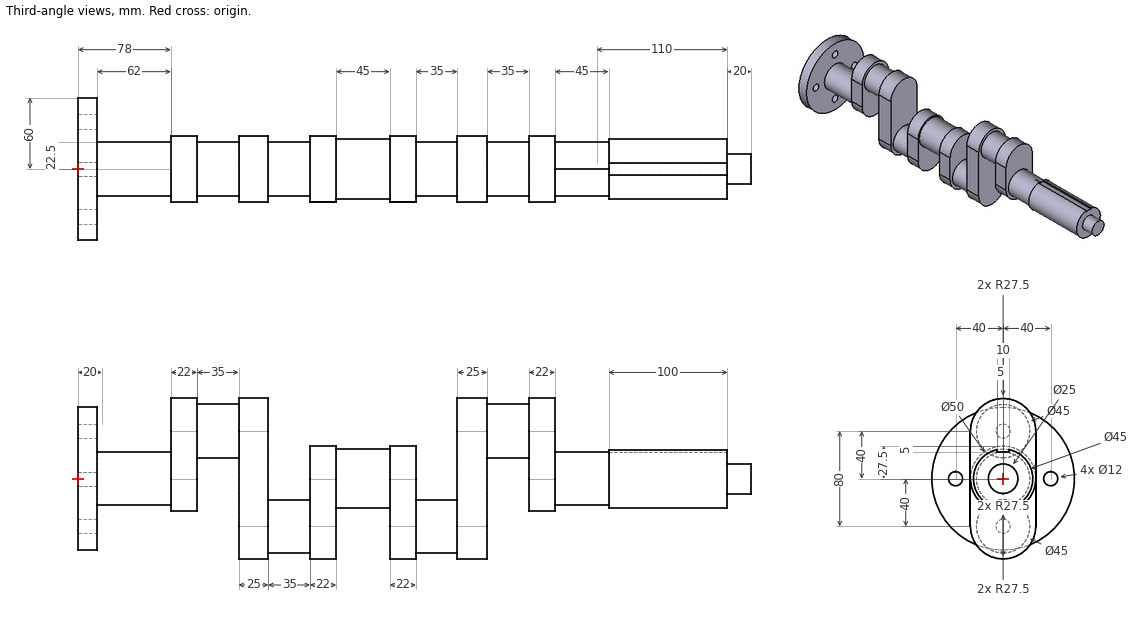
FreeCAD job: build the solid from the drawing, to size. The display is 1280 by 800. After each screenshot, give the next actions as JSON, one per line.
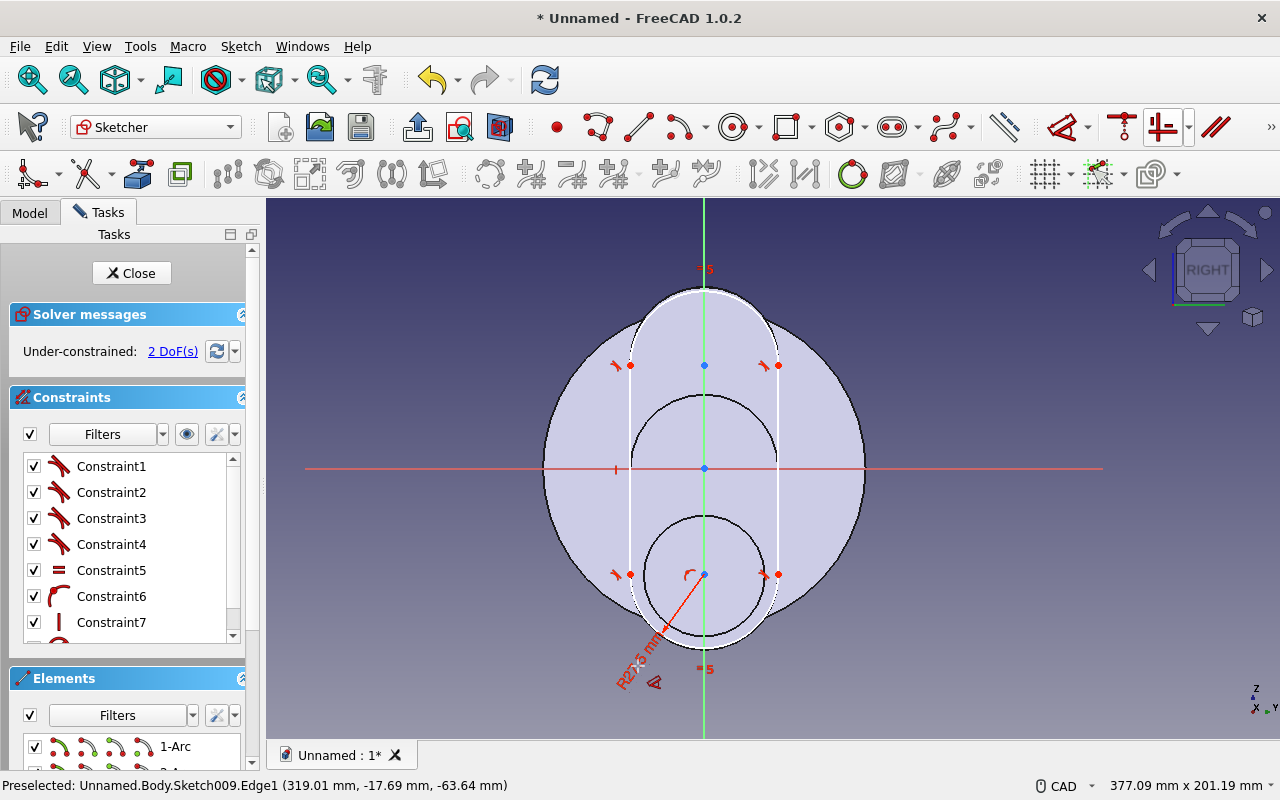
{"action": "left_click", "coordinate": [630, 511]}
{"action": "left_click", "coordinate": [596, 422]}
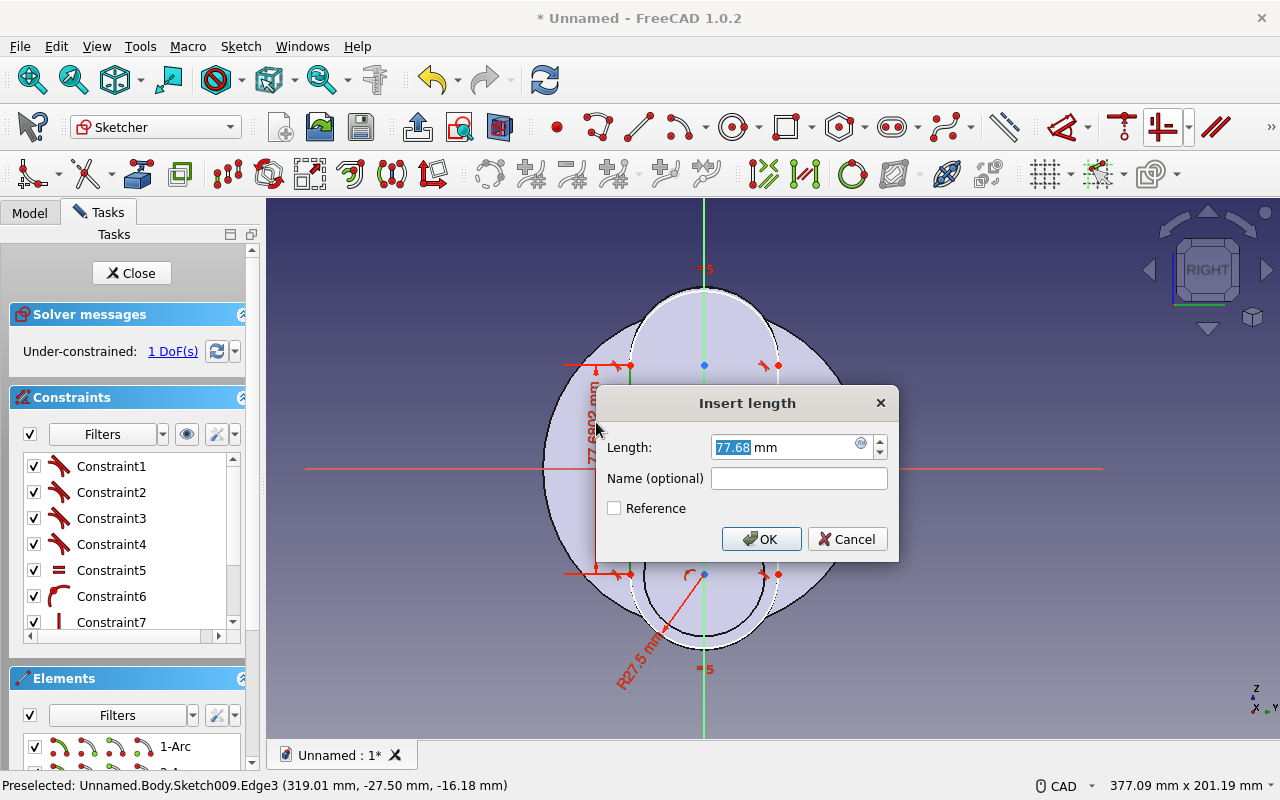
{"action": "type", "text": "80"}
{"action": "key", "text": "Return"}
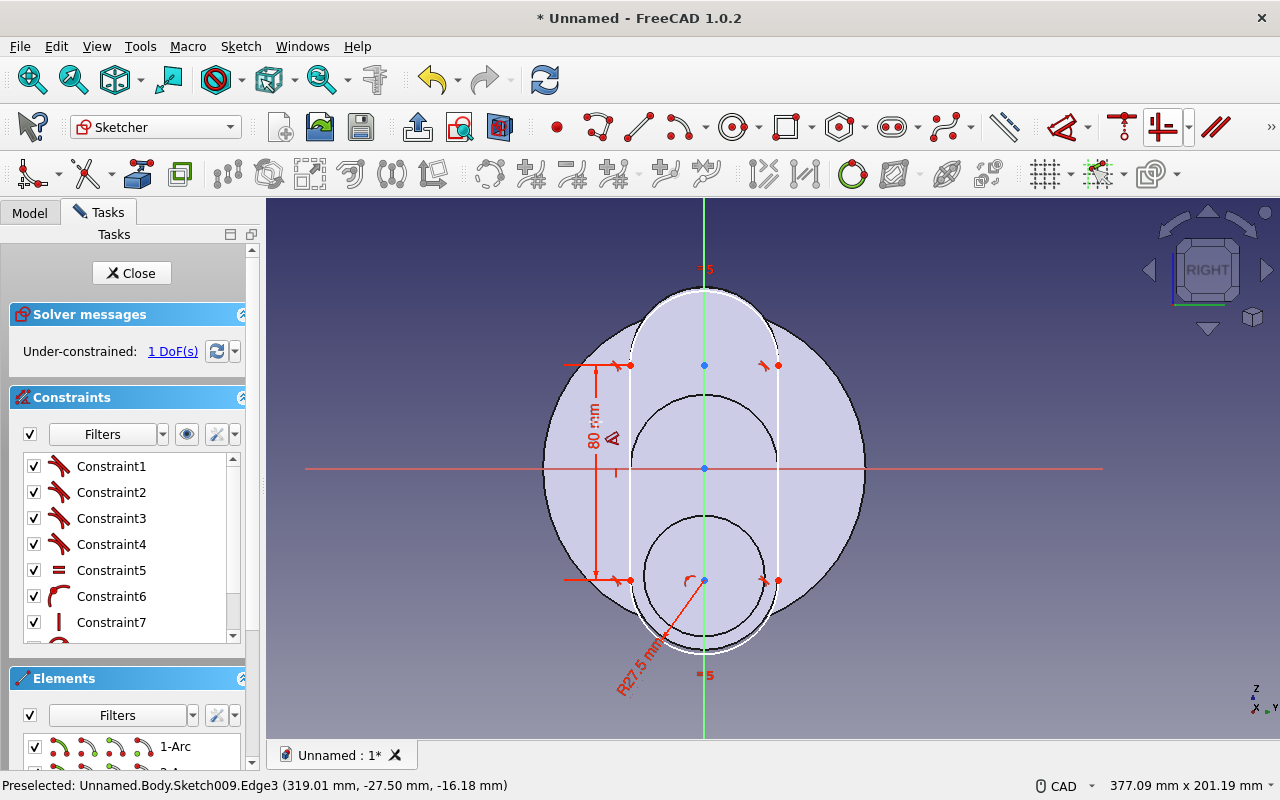
{"action": "left_click", "coordinate": [630, 580]}
{"action": "left_click", "coordinate": [596, 524]}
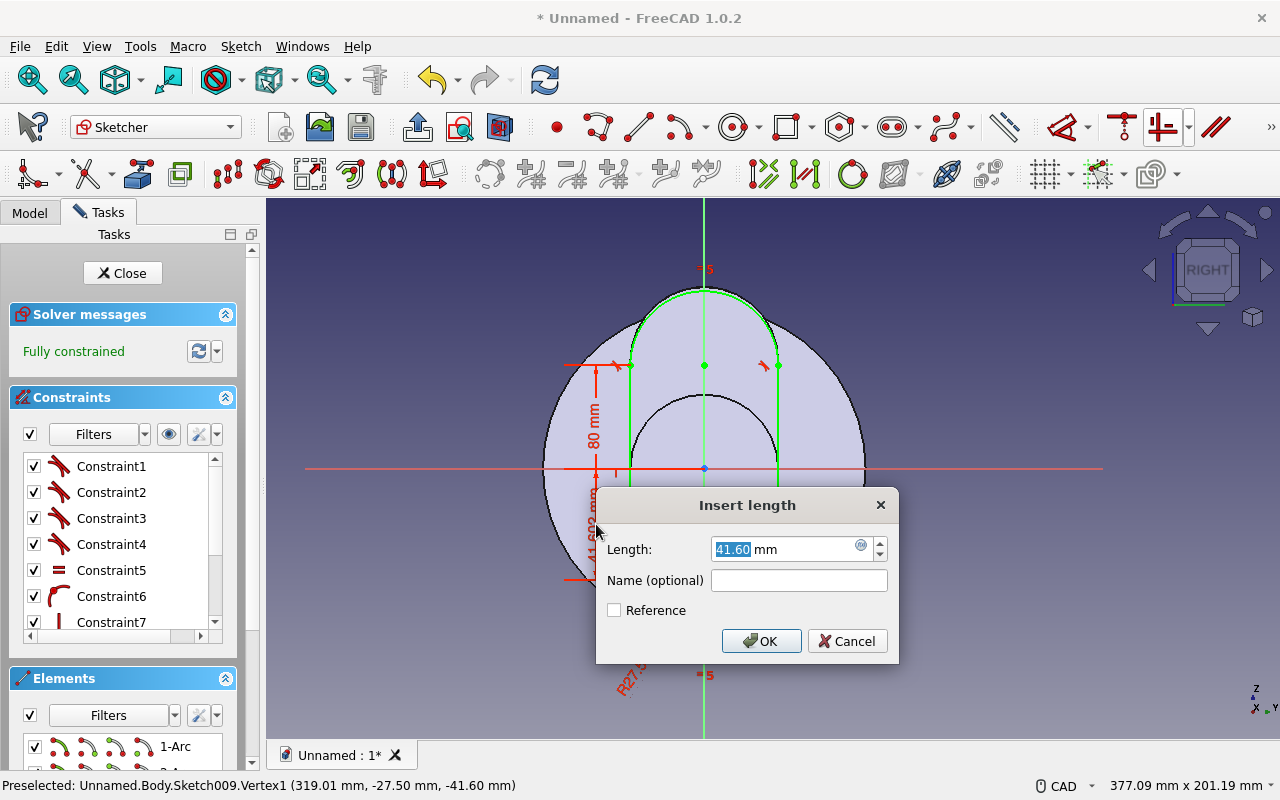
{"action": "type", "text": "40"}
{"action": "key", "text": "Return"}
{"action": "key", "text": "Escape"}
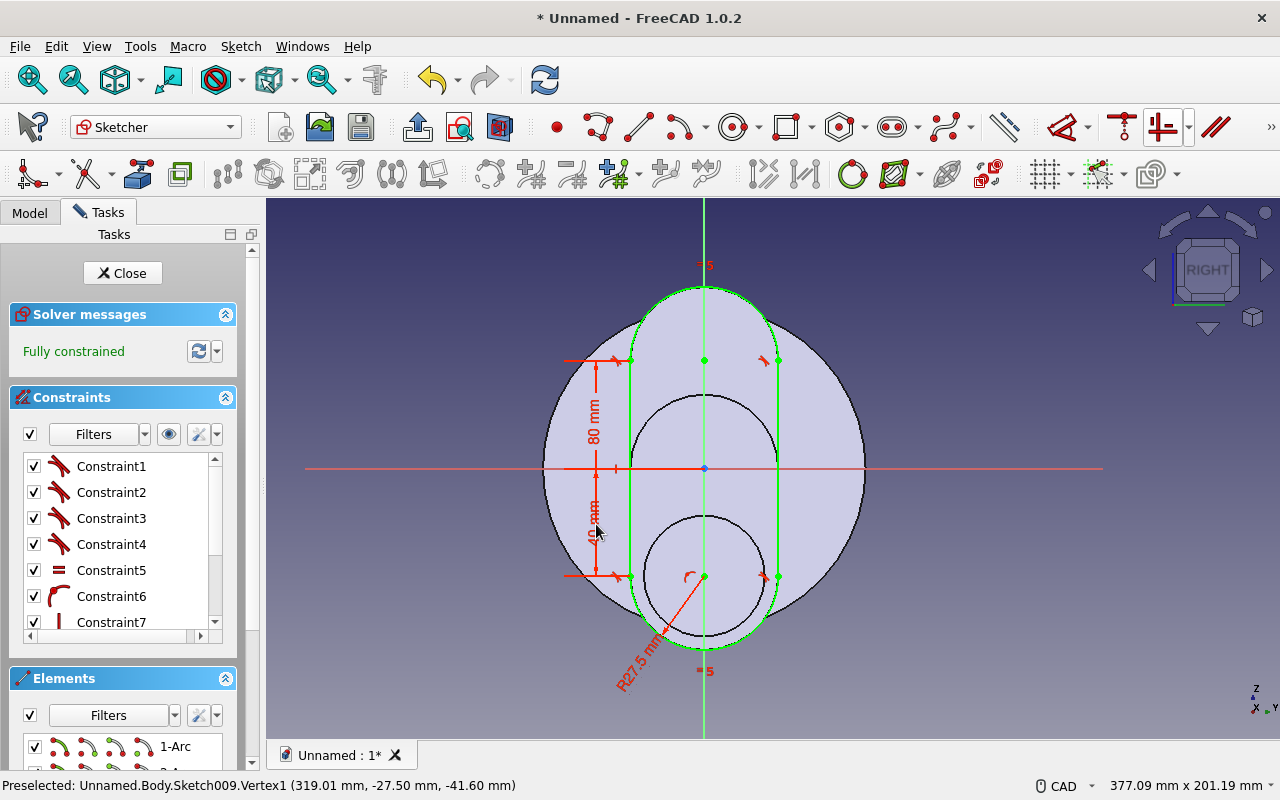
{"action": "left_click", "coordinate": [123, 273]}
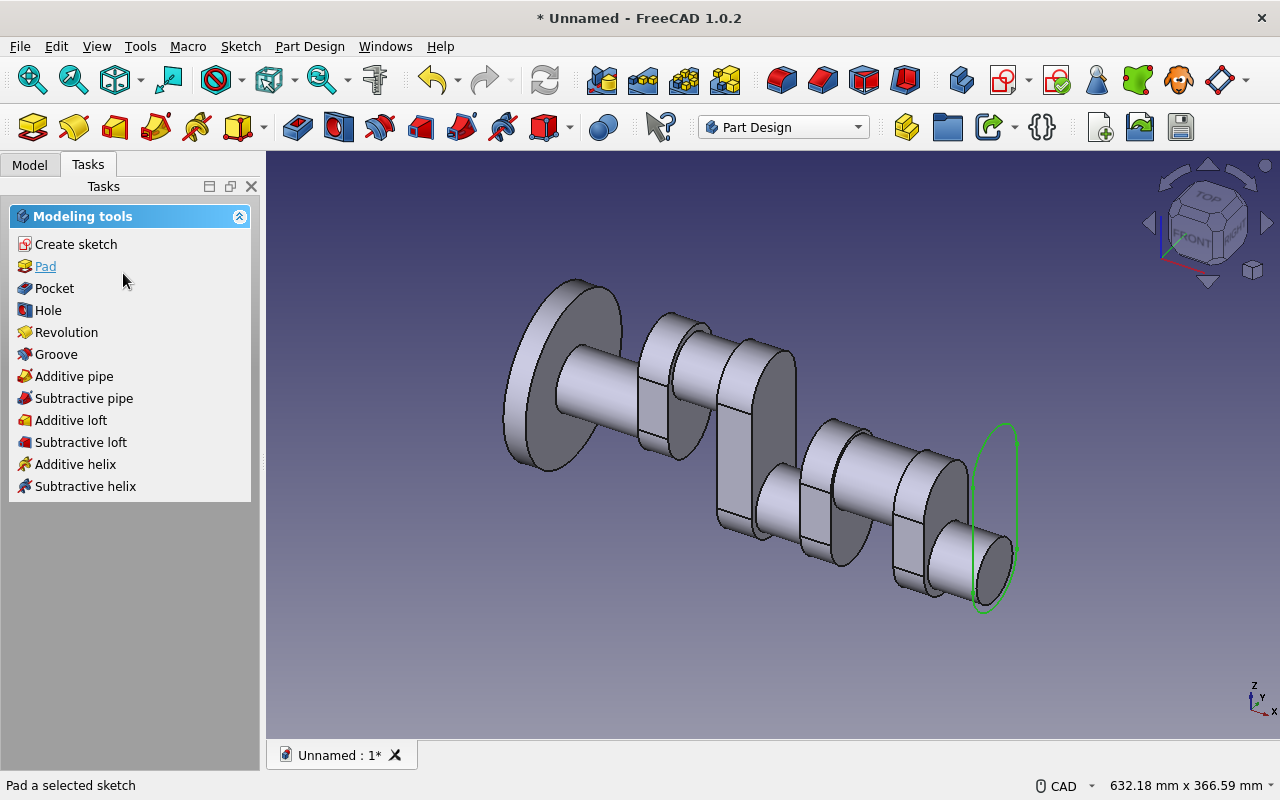
{"action": "left_click", "coordinate": [33, 128]}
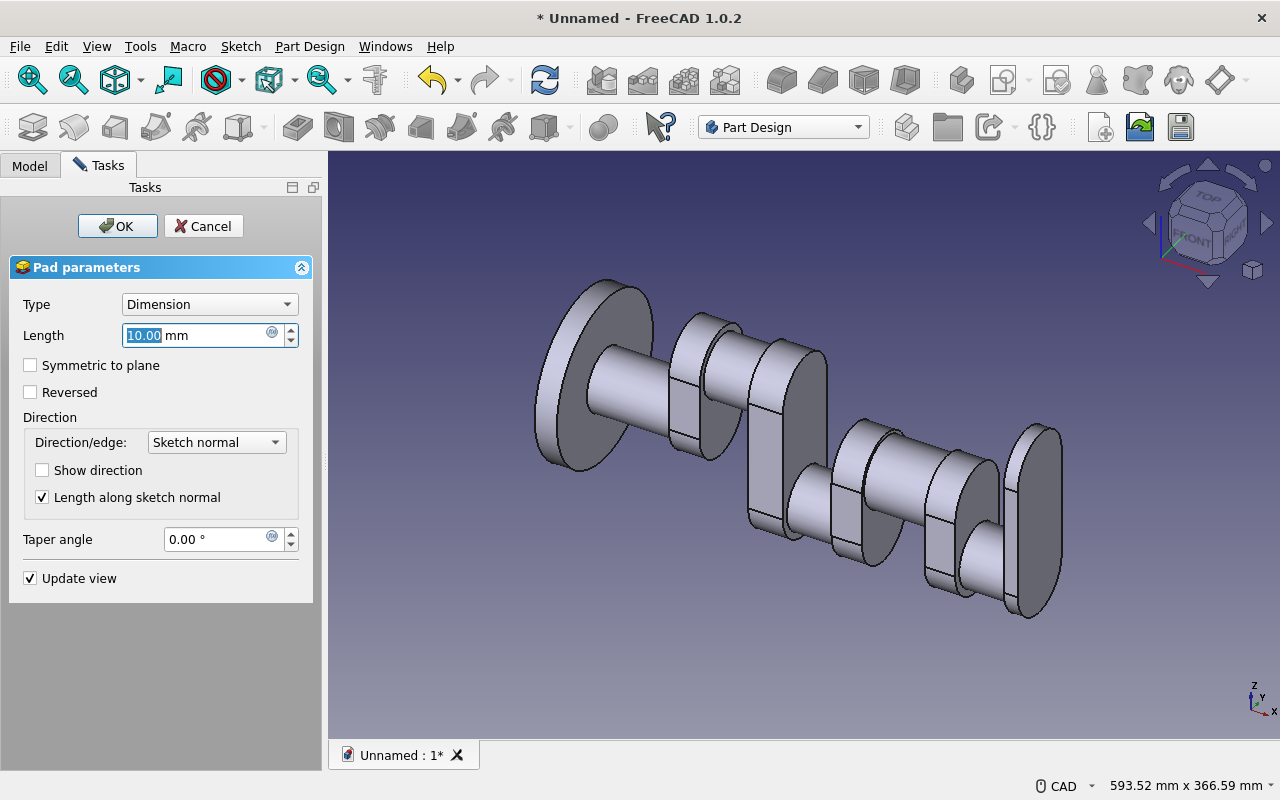
{"action": "type", "text": "25"}
{"action": "key", "text": "Tab"}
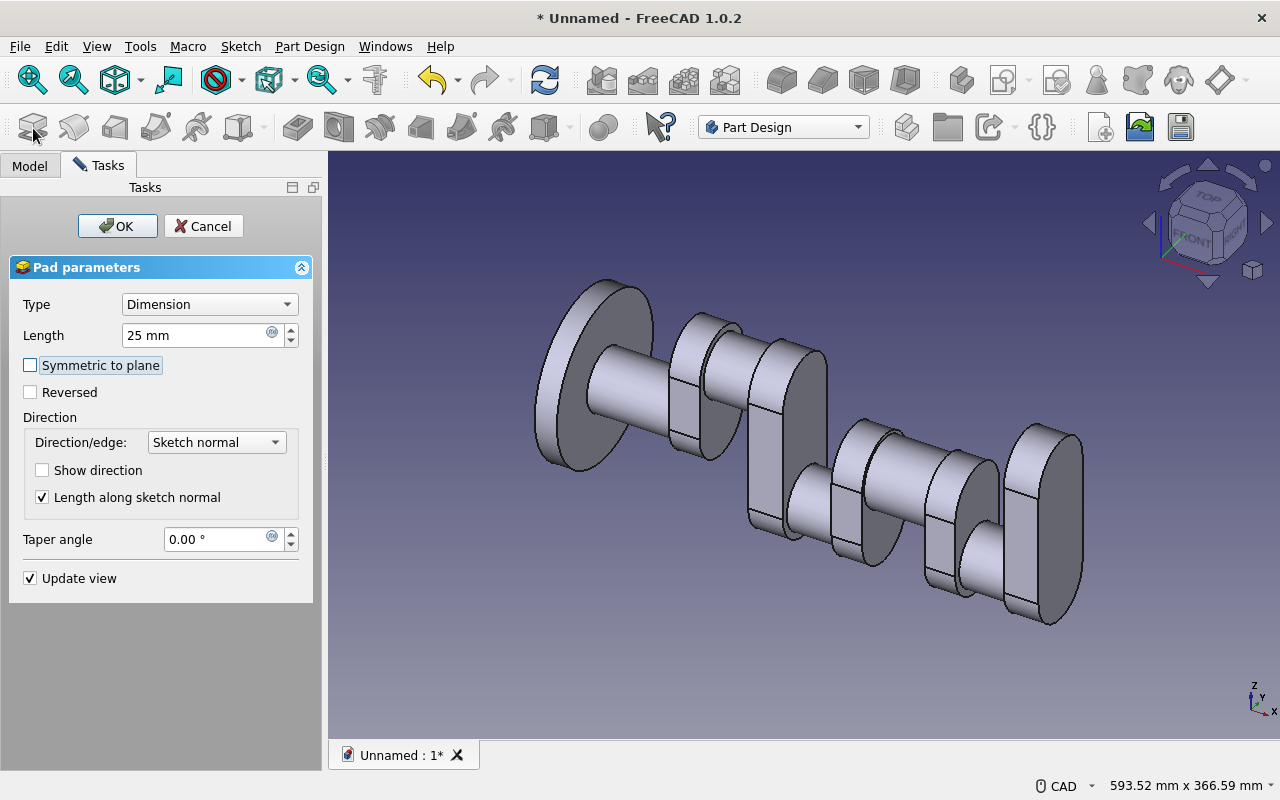
{"action": "left_click", "coordinate": [118, 226]}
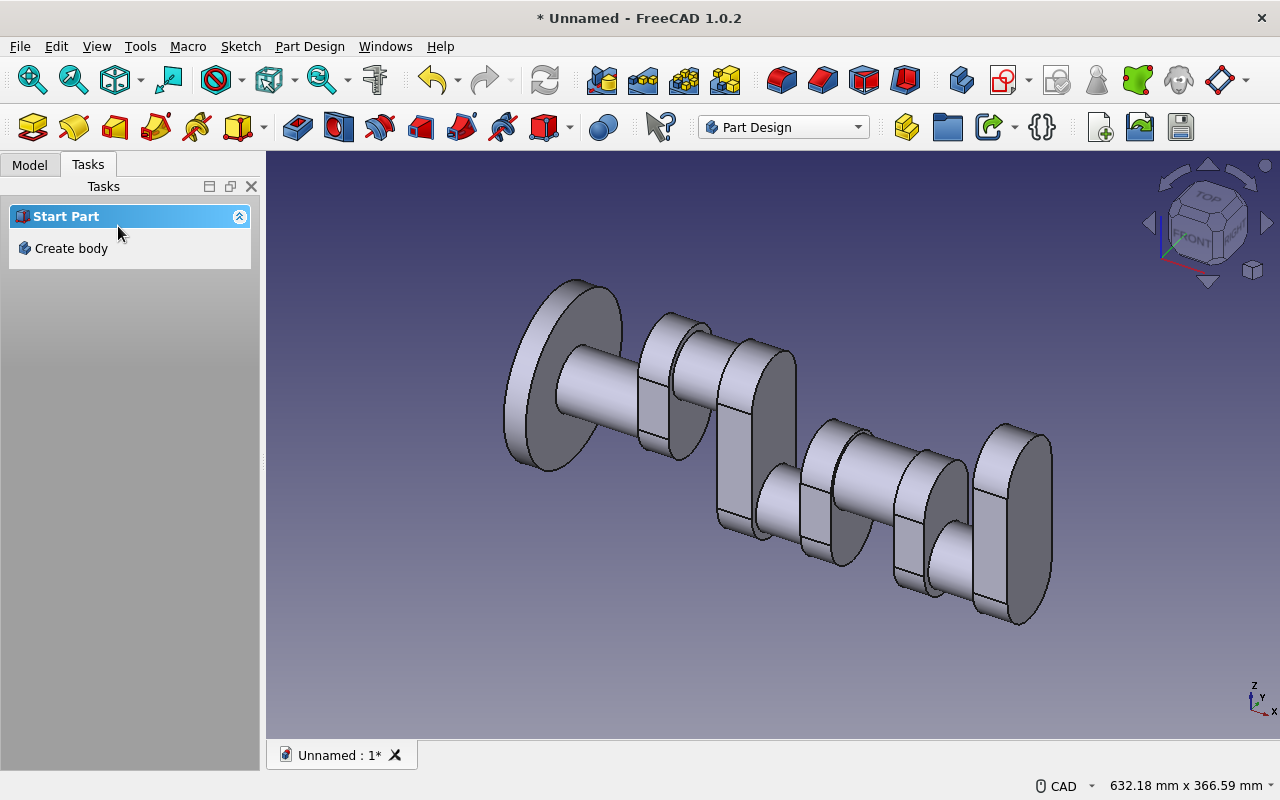
{"action": "left_click", "coordinate": [1030, 478]}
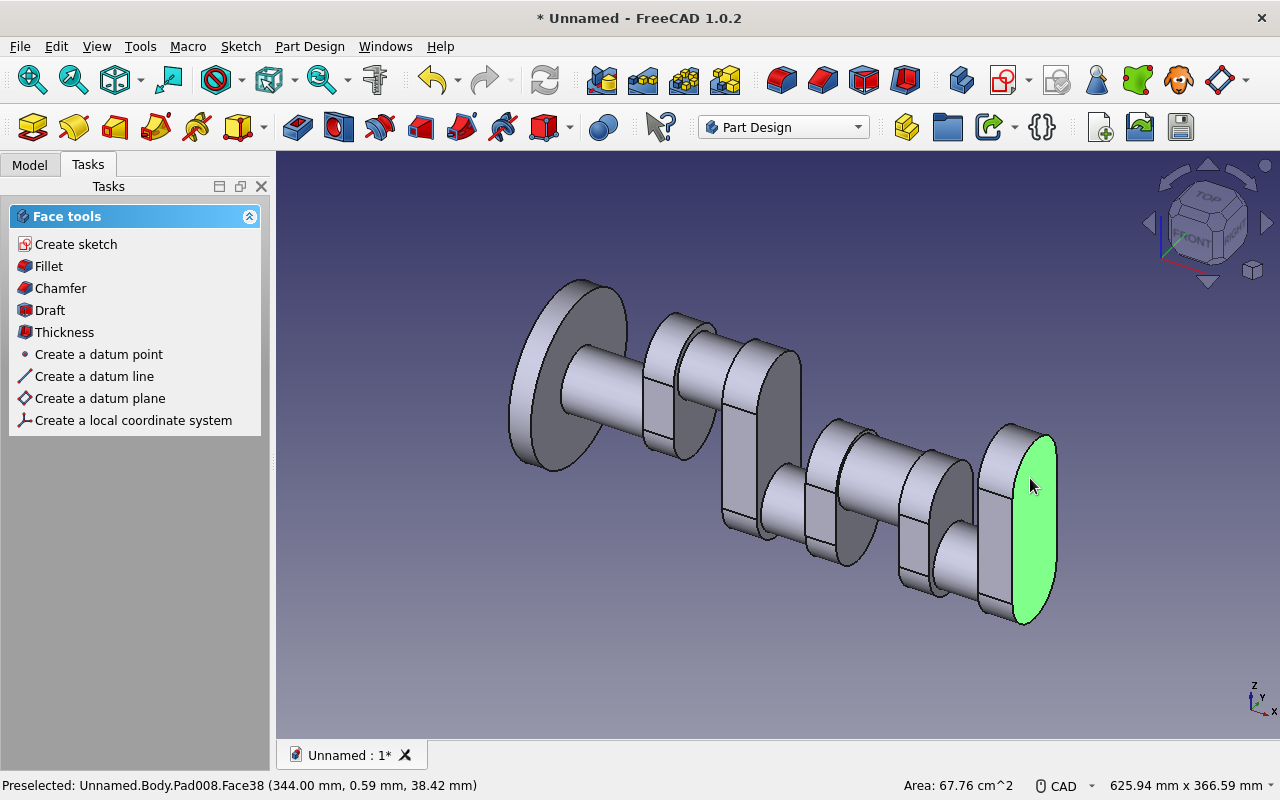
{"action": "left_click", "coordinate": [1002, 80]}